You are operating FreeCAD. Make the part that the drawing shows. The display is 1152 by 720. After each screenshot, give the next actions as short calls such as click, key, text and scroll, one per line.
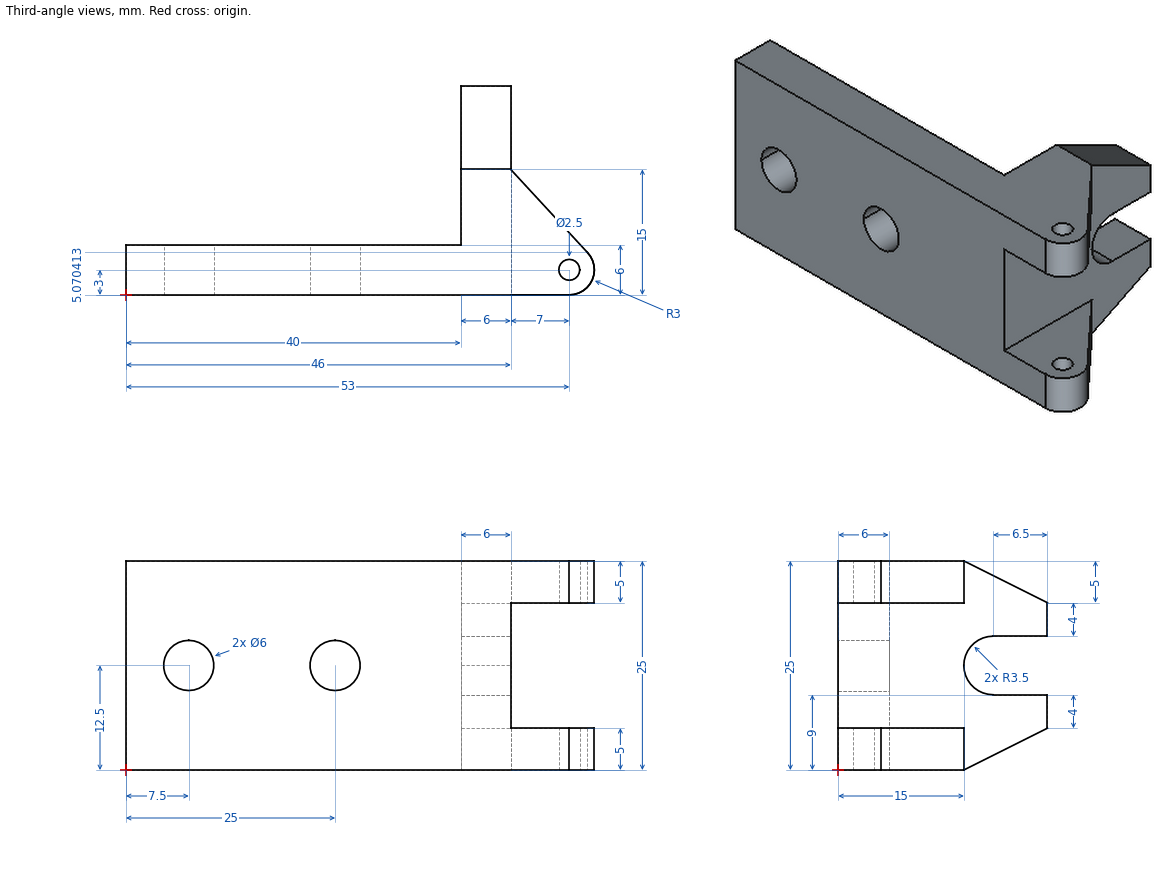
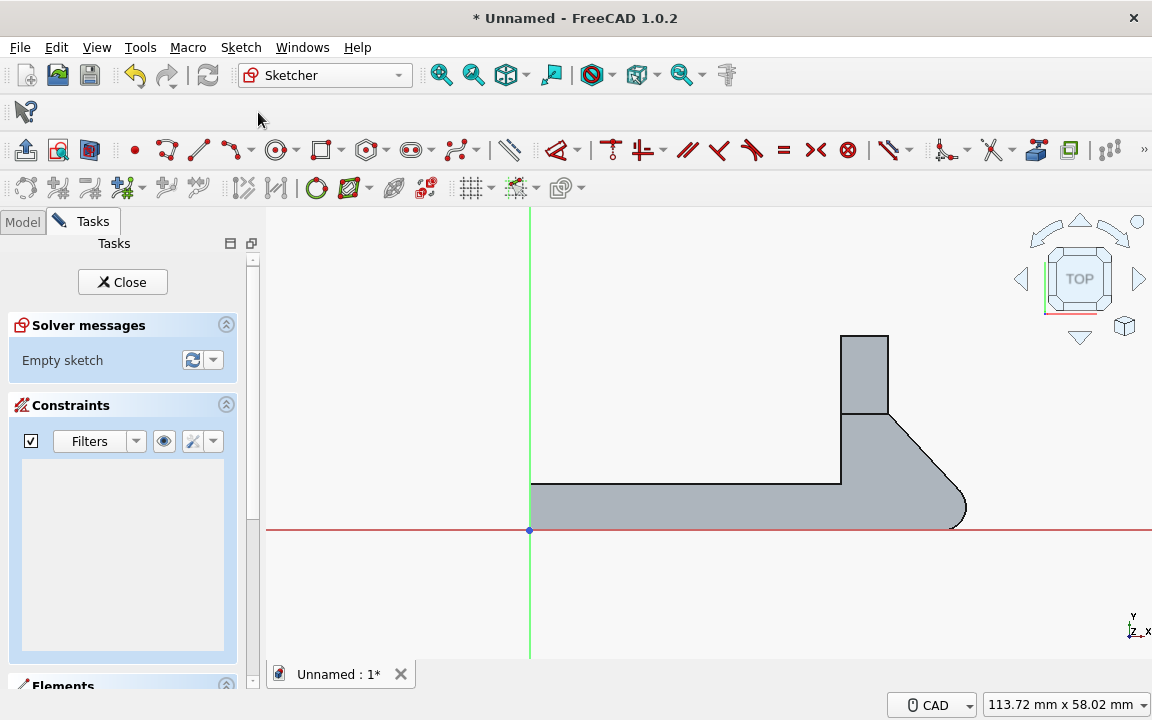
scroll(967, 513, up, 13)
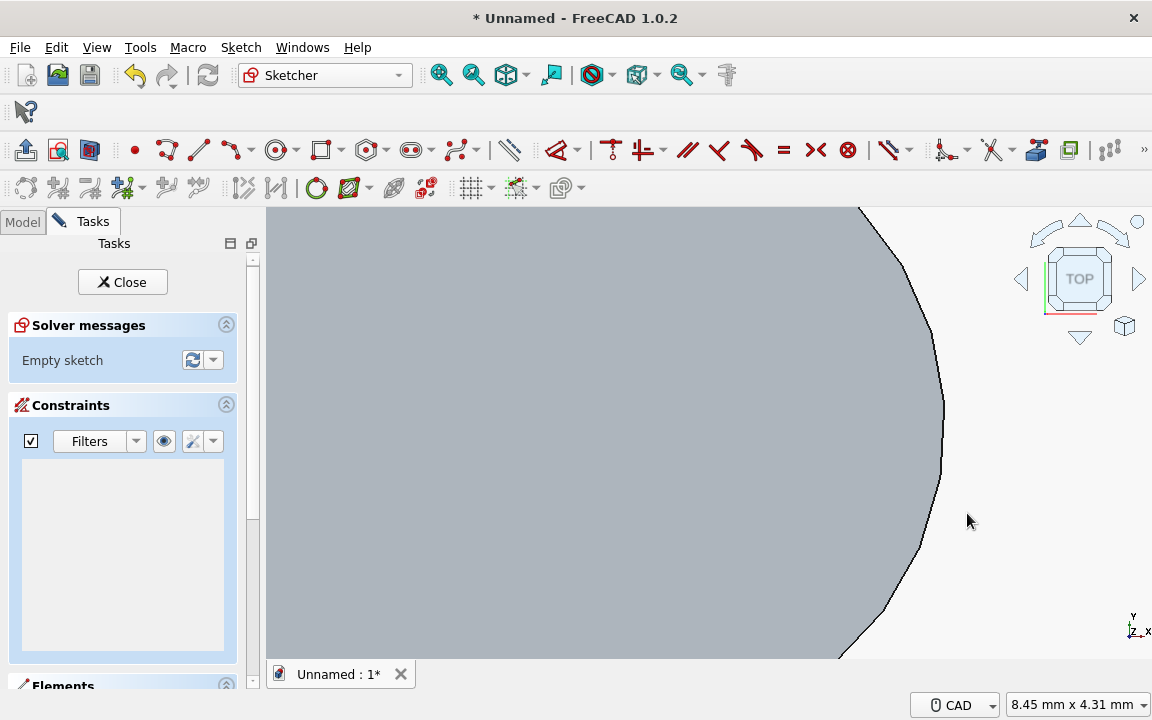
click(276, 150)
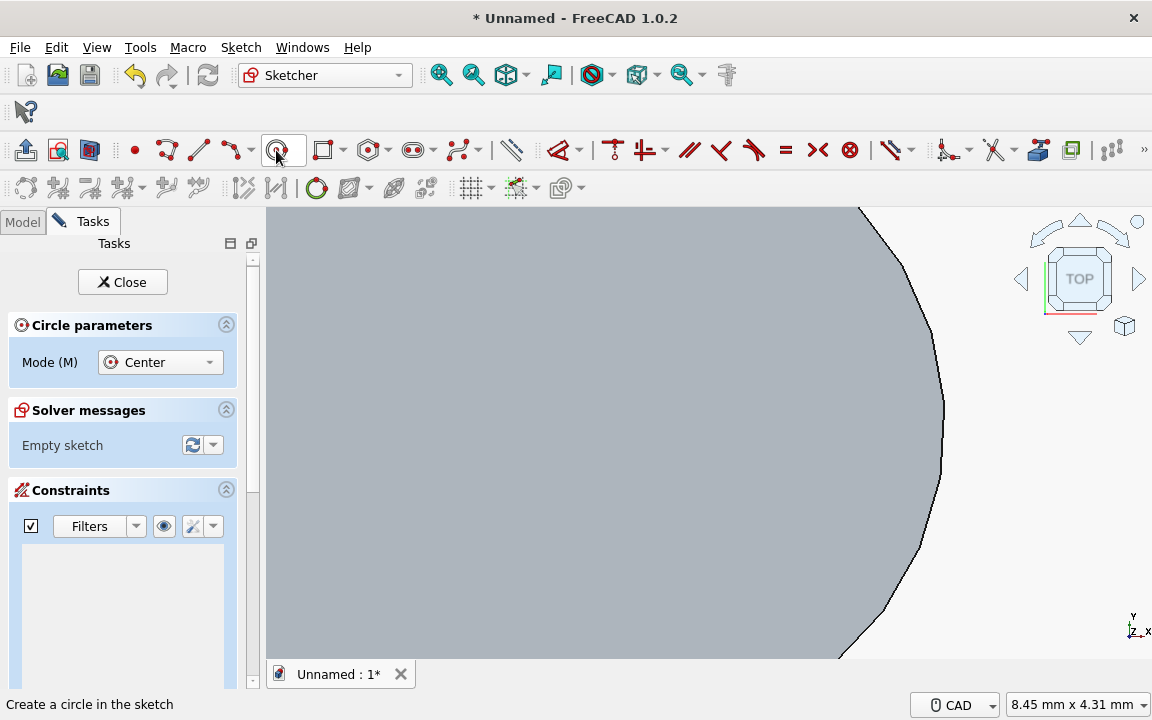
click(630, 424)
click(723, 331)
key(Escape)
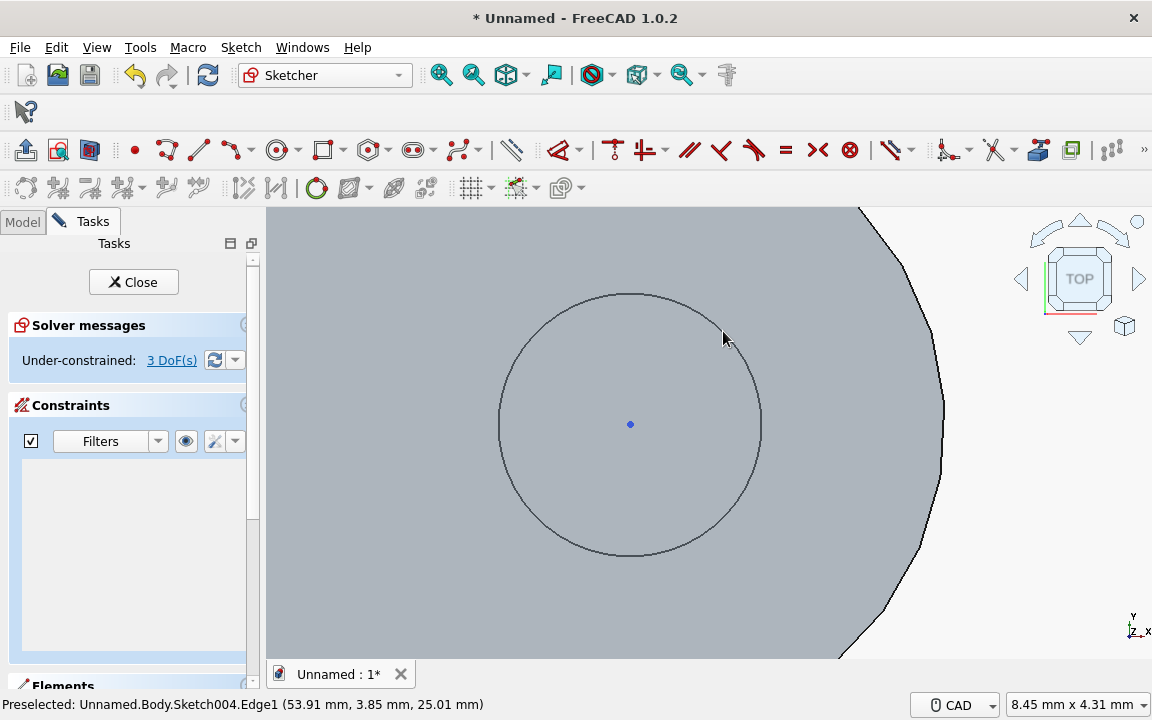
key(d)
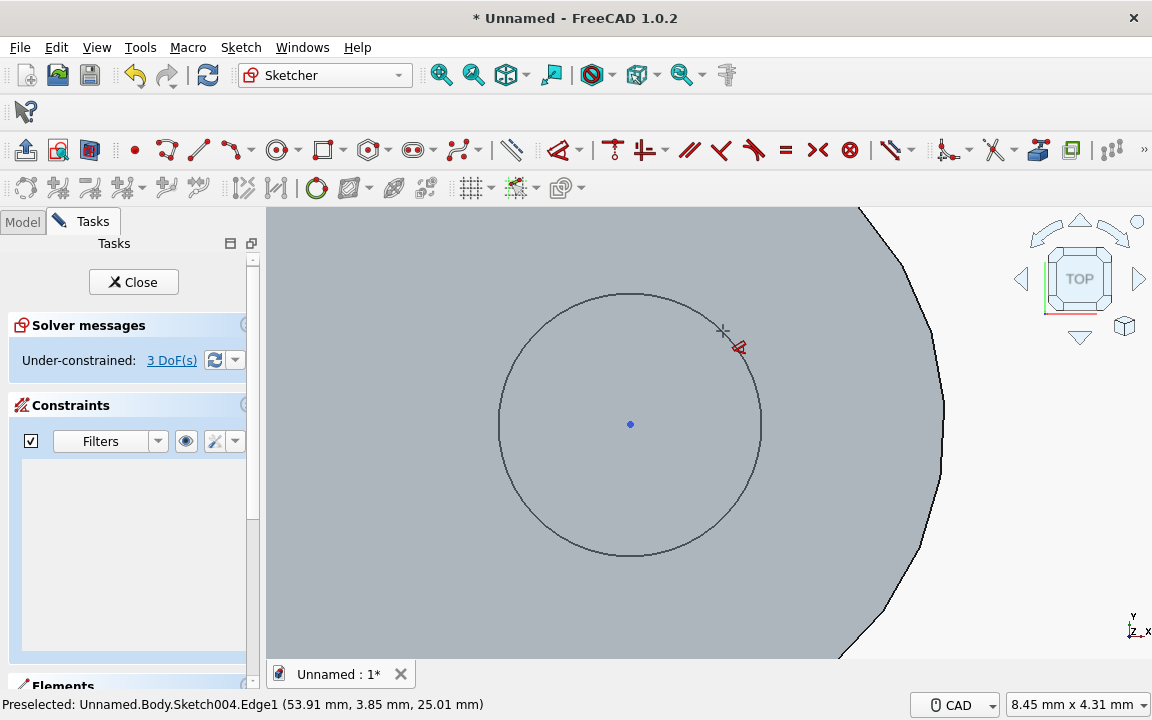
click(723, 332)
click(746, 309)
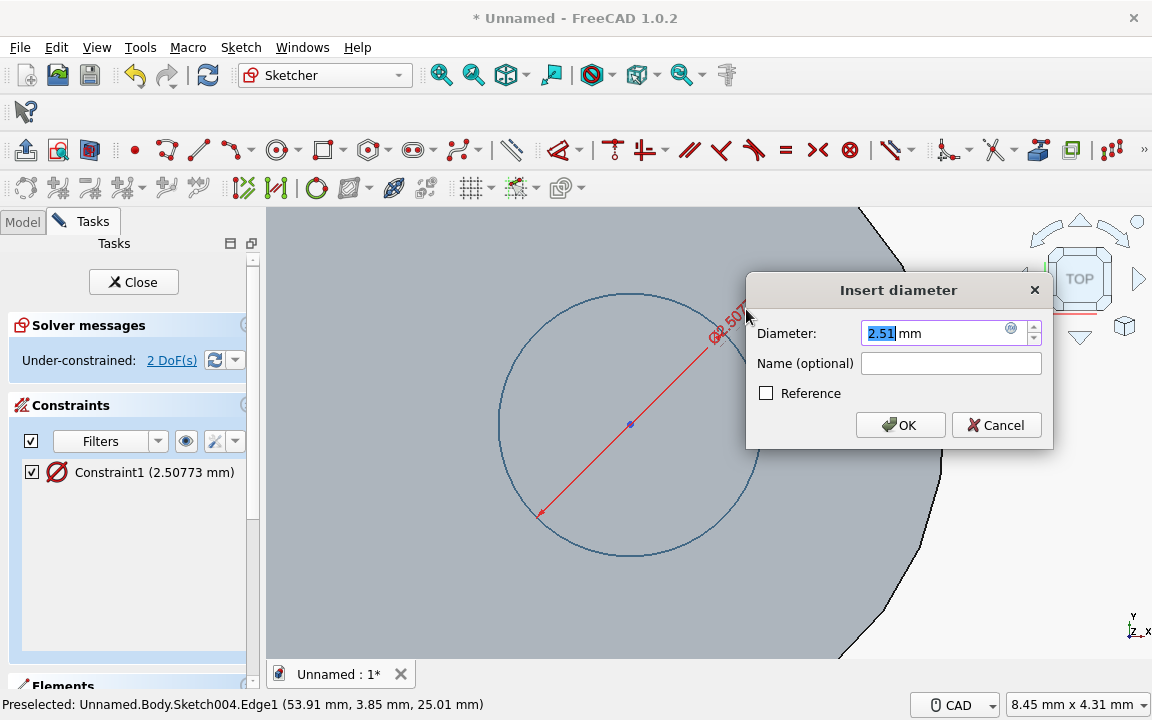
text(2.5)
key(Return)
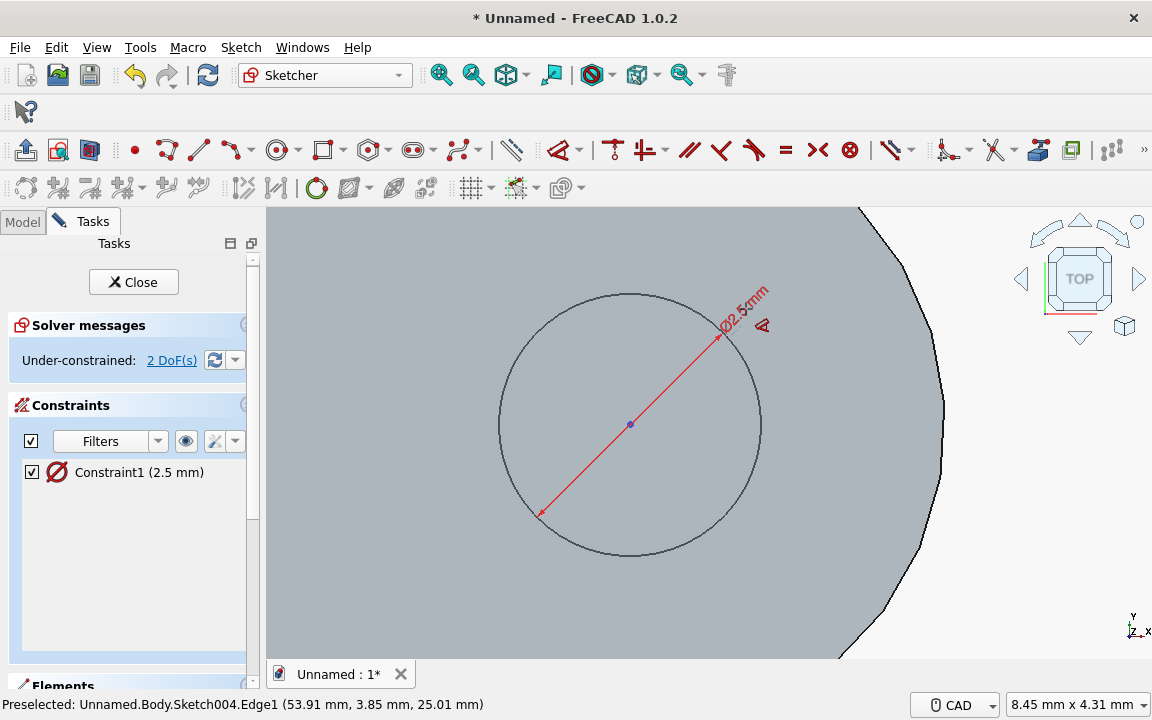
click(630, 425)
click(664, 528)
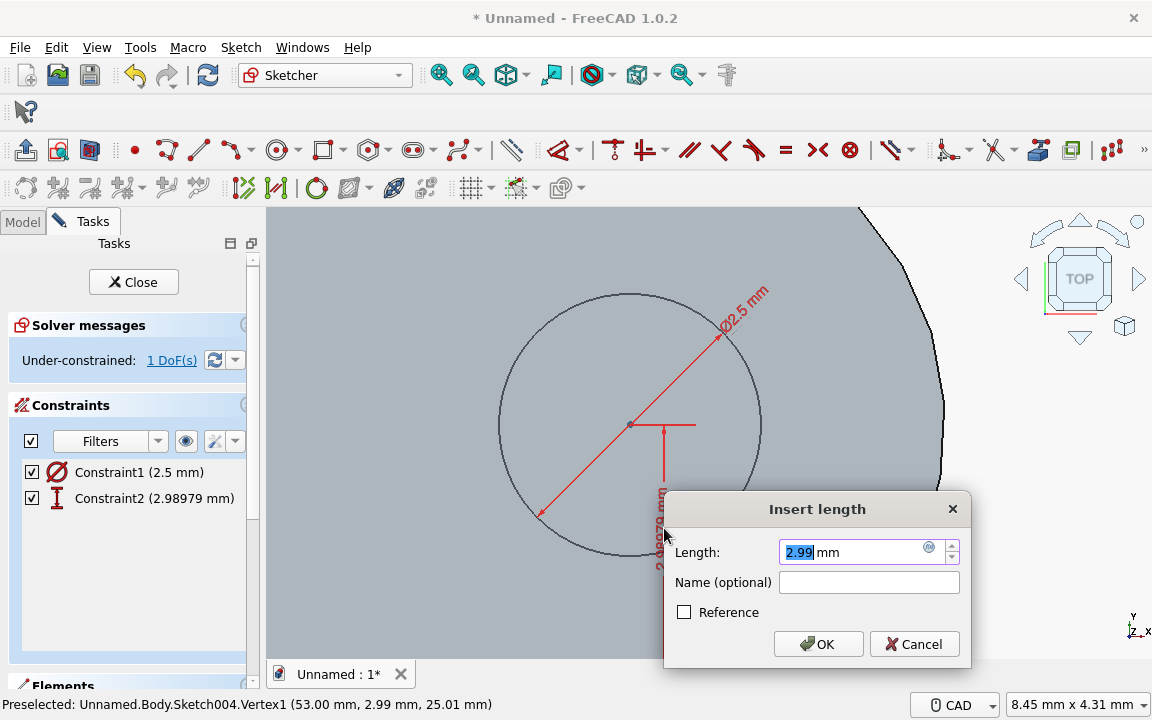
text(3)
key(Return)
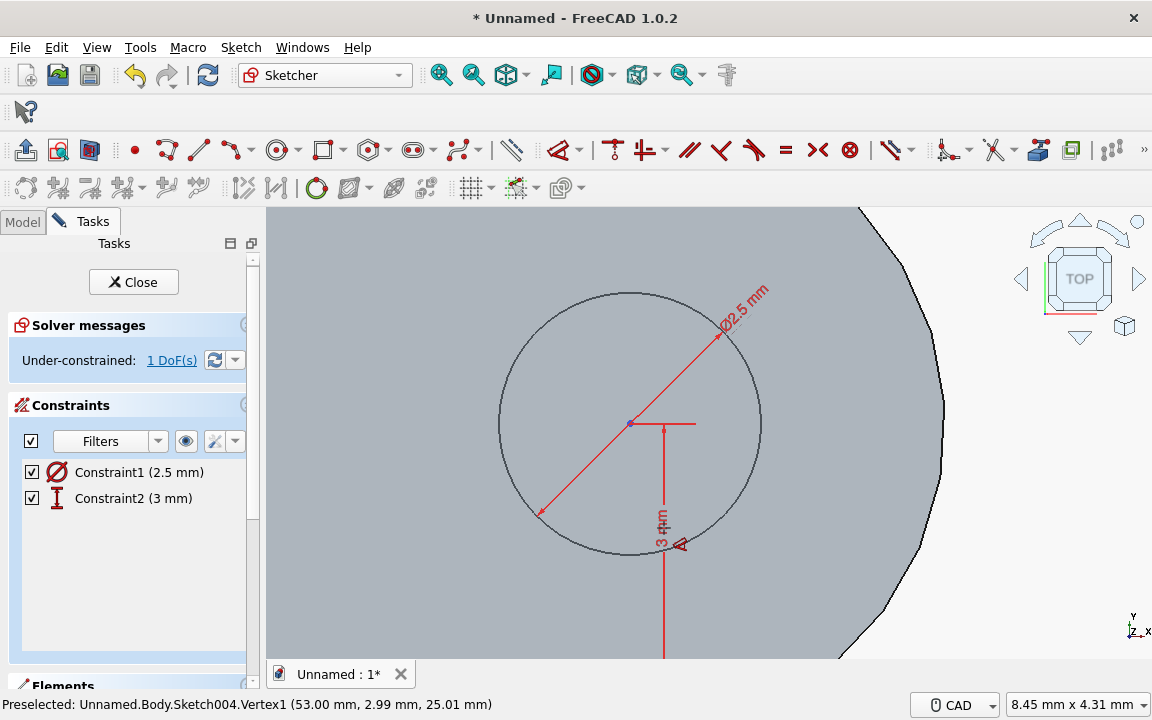
click(630, 424)
click(462, 390)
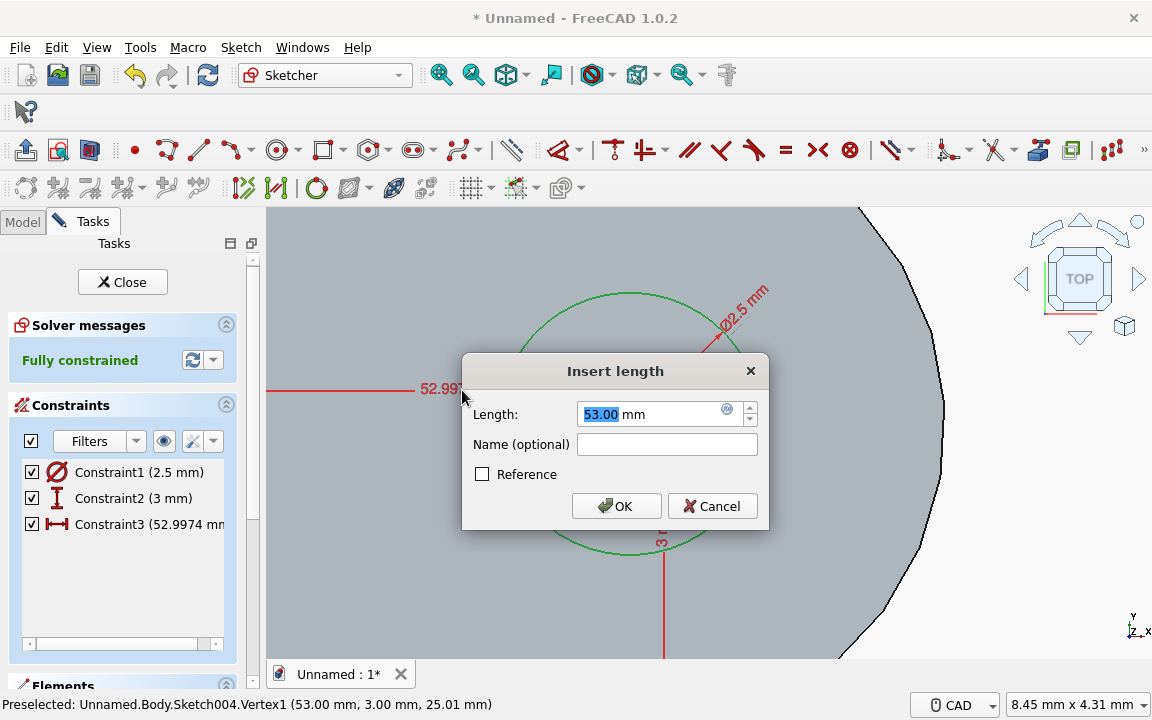
text(53)
key(Return)
key(Escape)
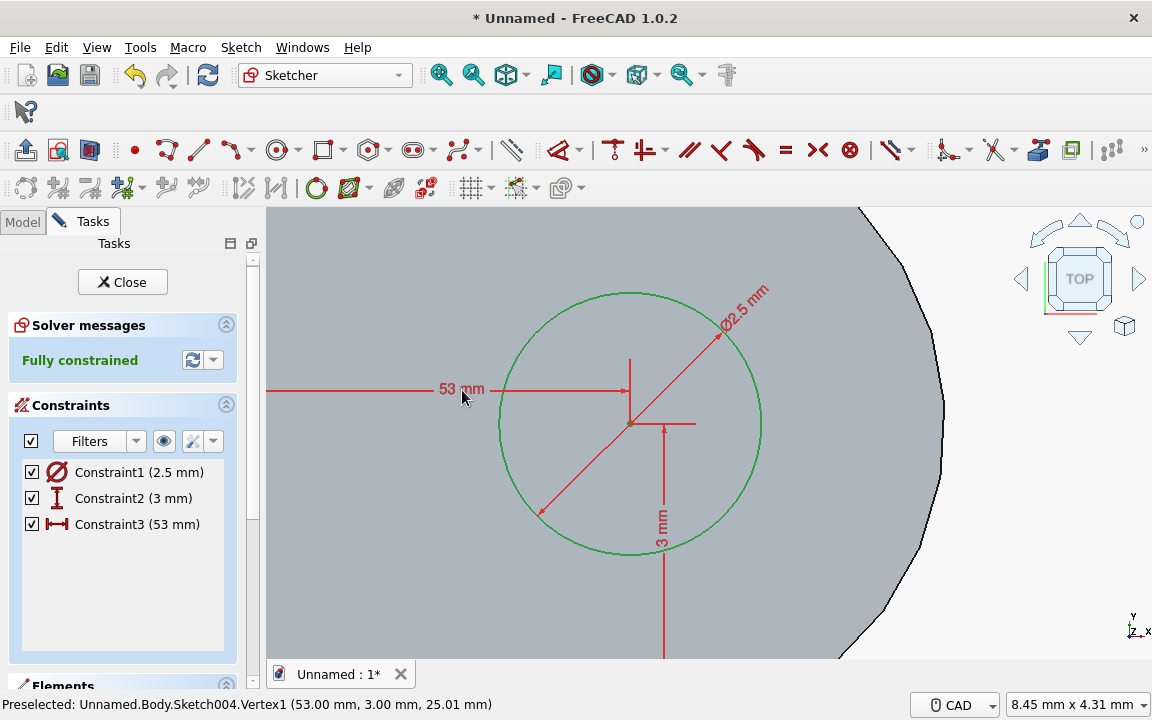
click(123, 282)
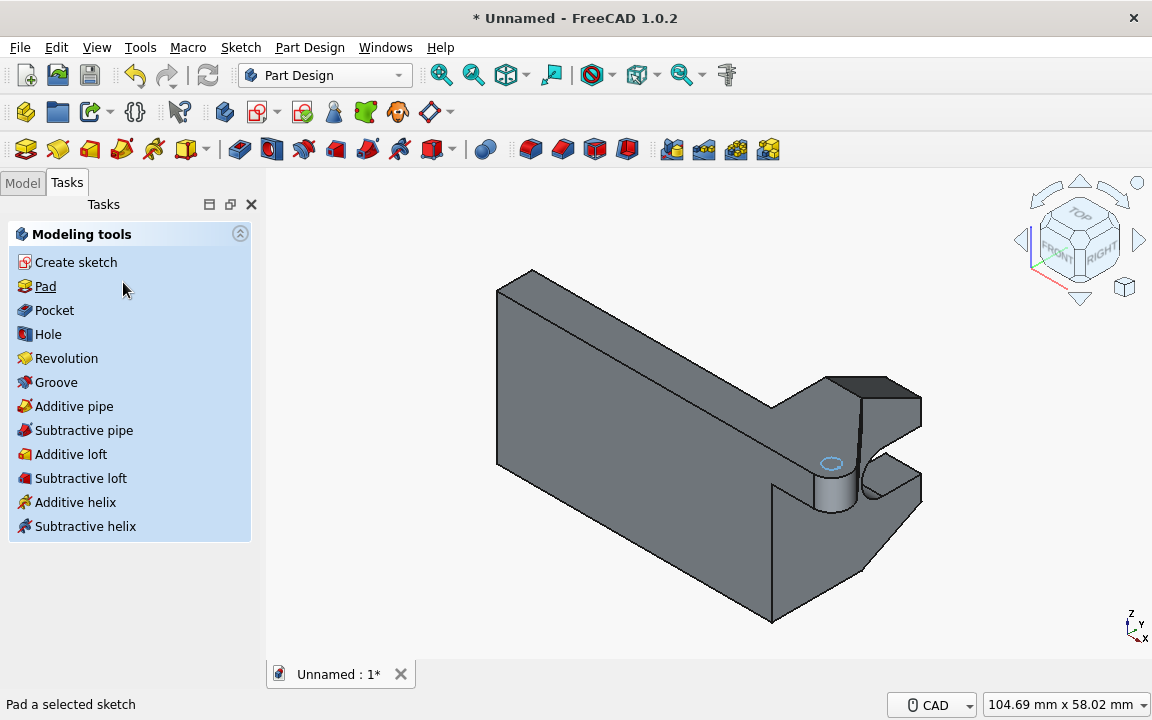
click(240, 150)